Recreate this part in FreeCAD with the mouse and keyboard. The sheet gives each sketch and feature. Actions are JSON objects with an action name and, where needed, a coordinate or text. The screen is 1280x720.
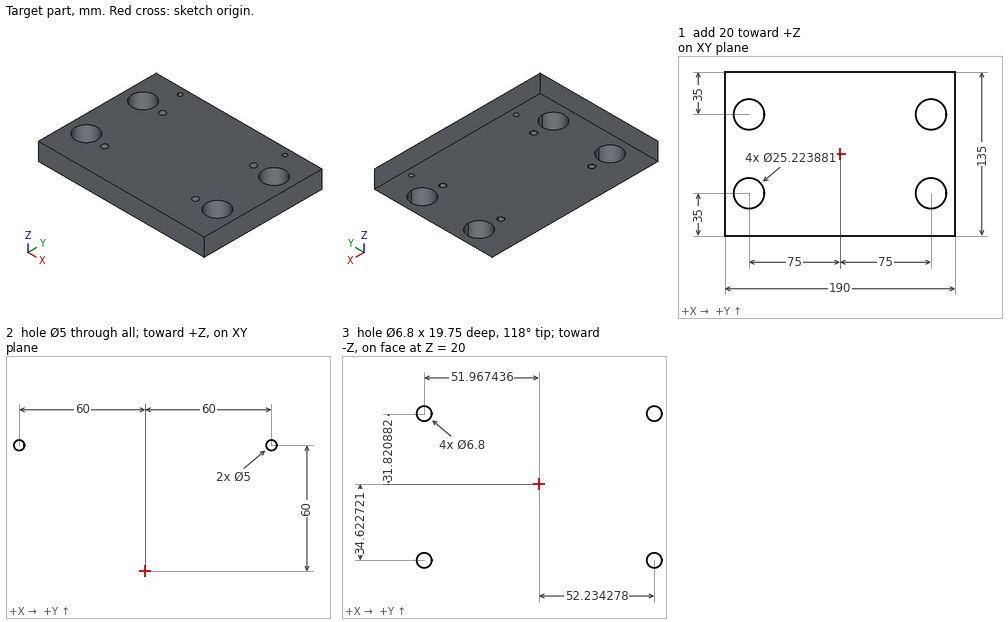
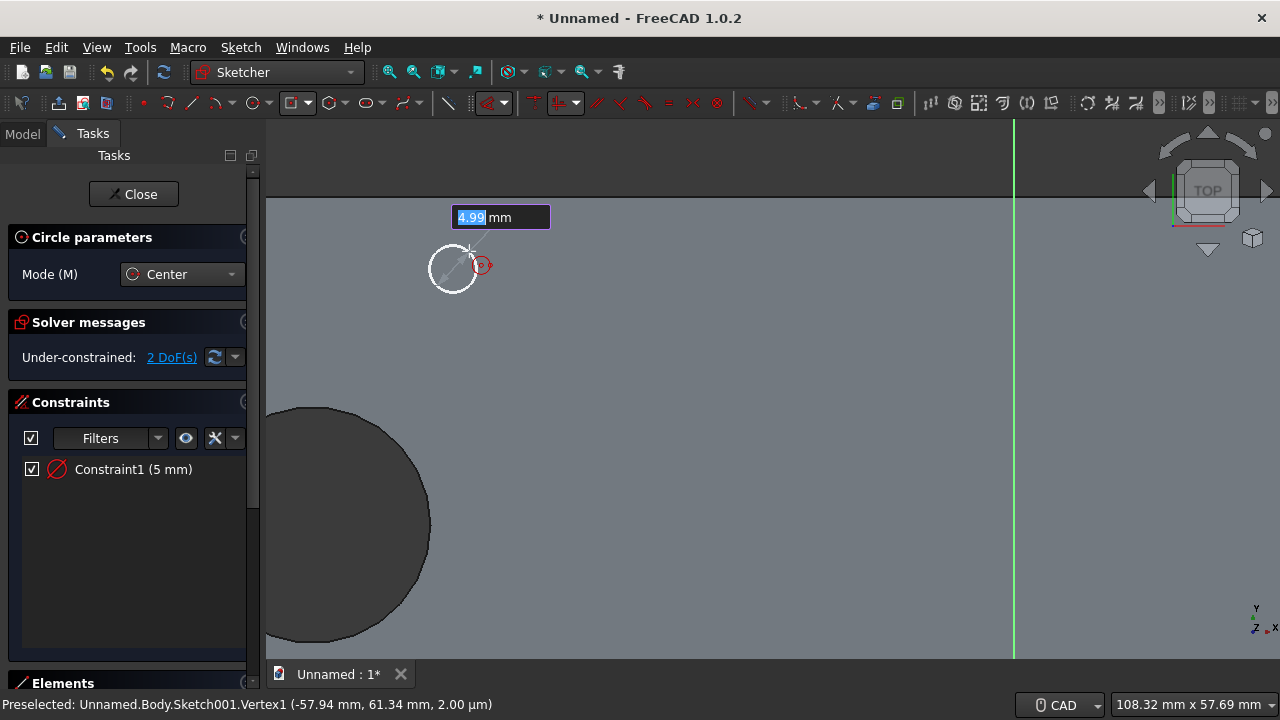
{"action": "type", "text": "5"}
{"action": "key", "text": "Return"}
{"action": "key", "text": "Escape"}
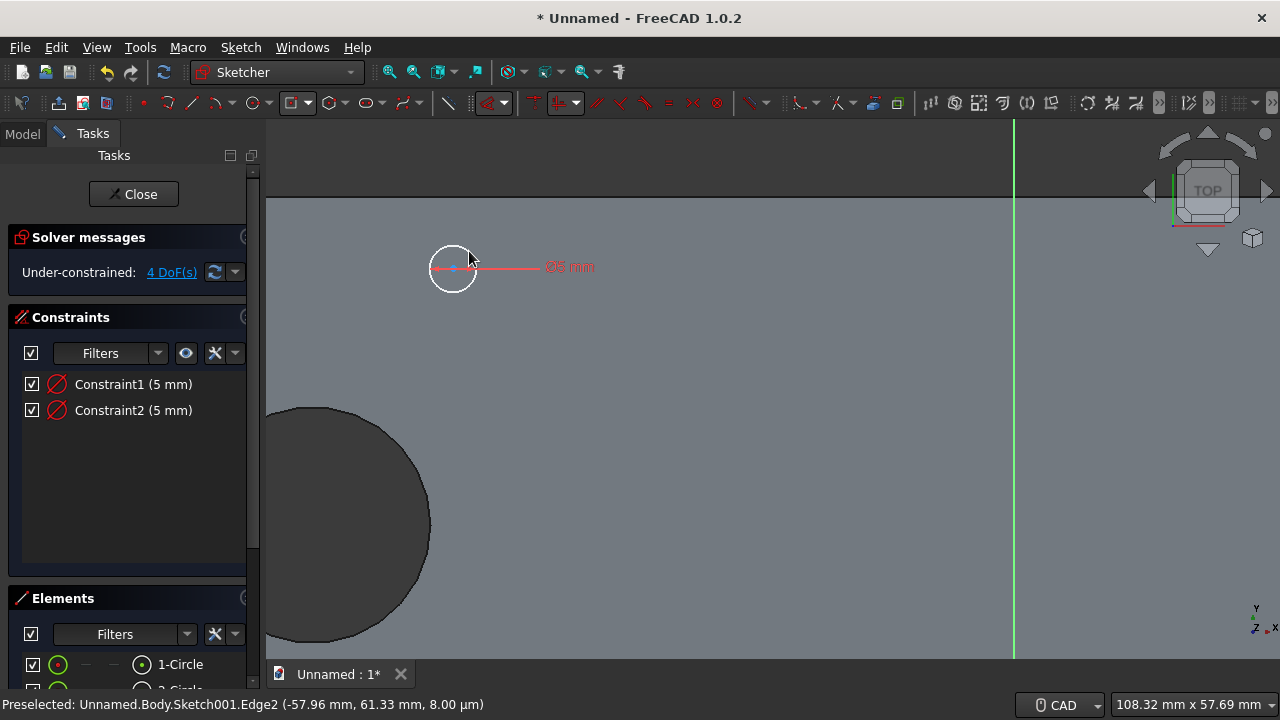
{"action": "scroll", "coordinate": [452, 268], "scroll_direction": "down", "scroll_amount": 4}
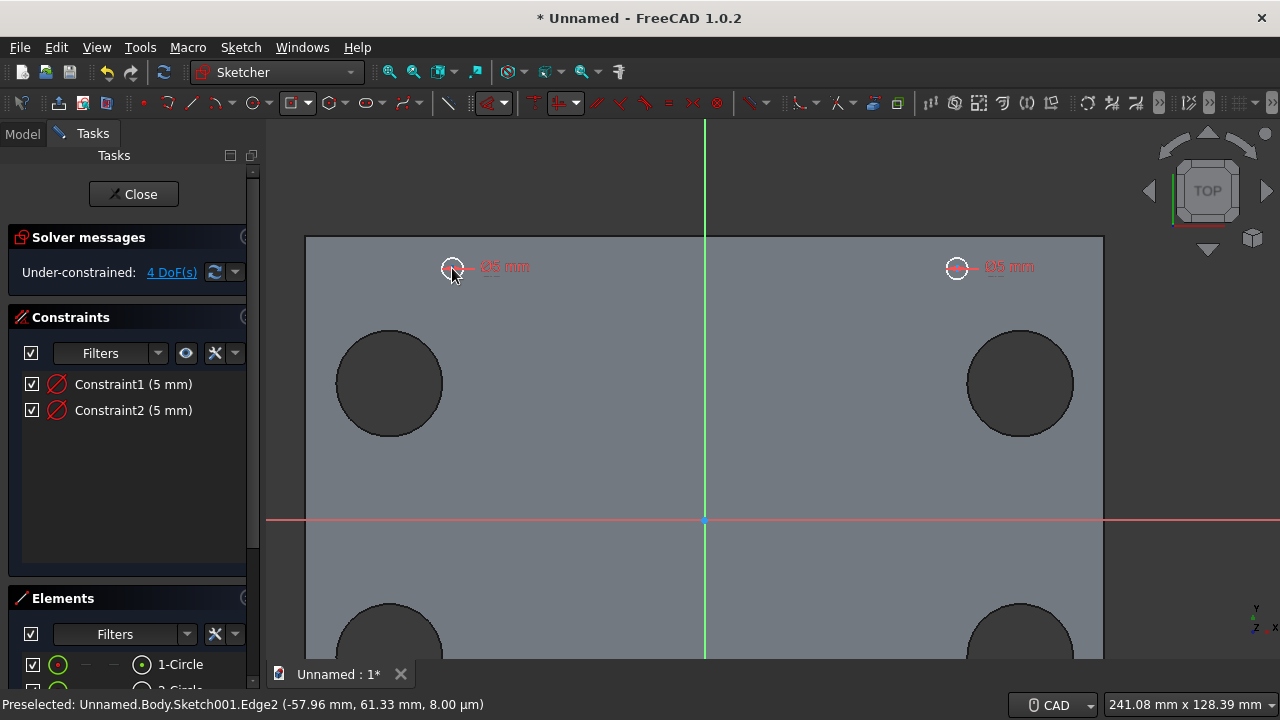
{"action": "left_click", "coordinate": [957, 269]}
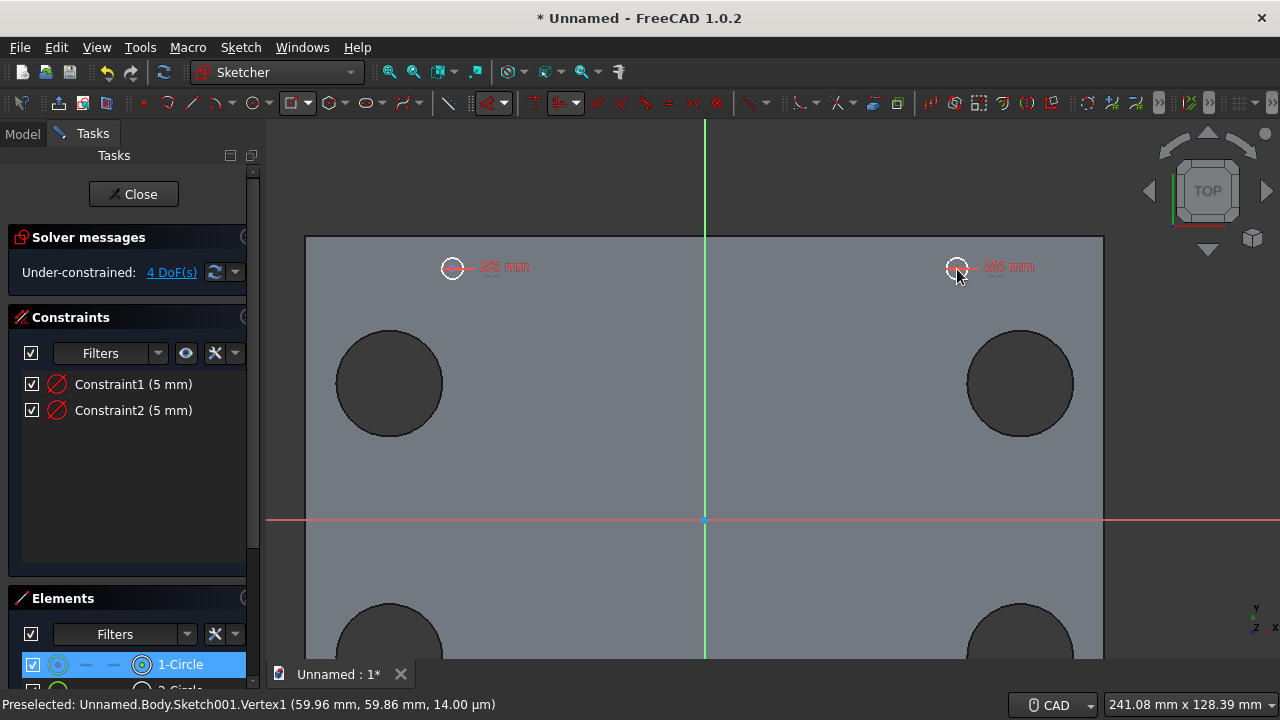
{"action": "left_click", "coordinate": [453, 269]}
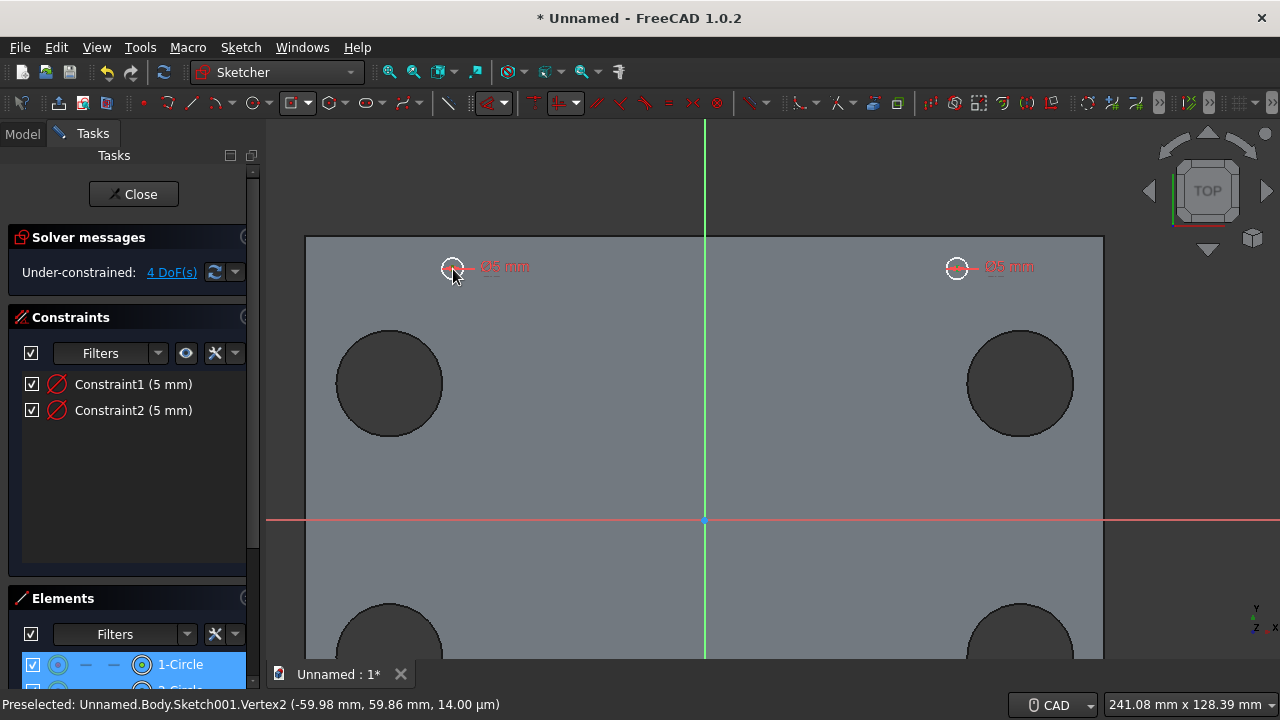
{"action": "key", "text": "h"}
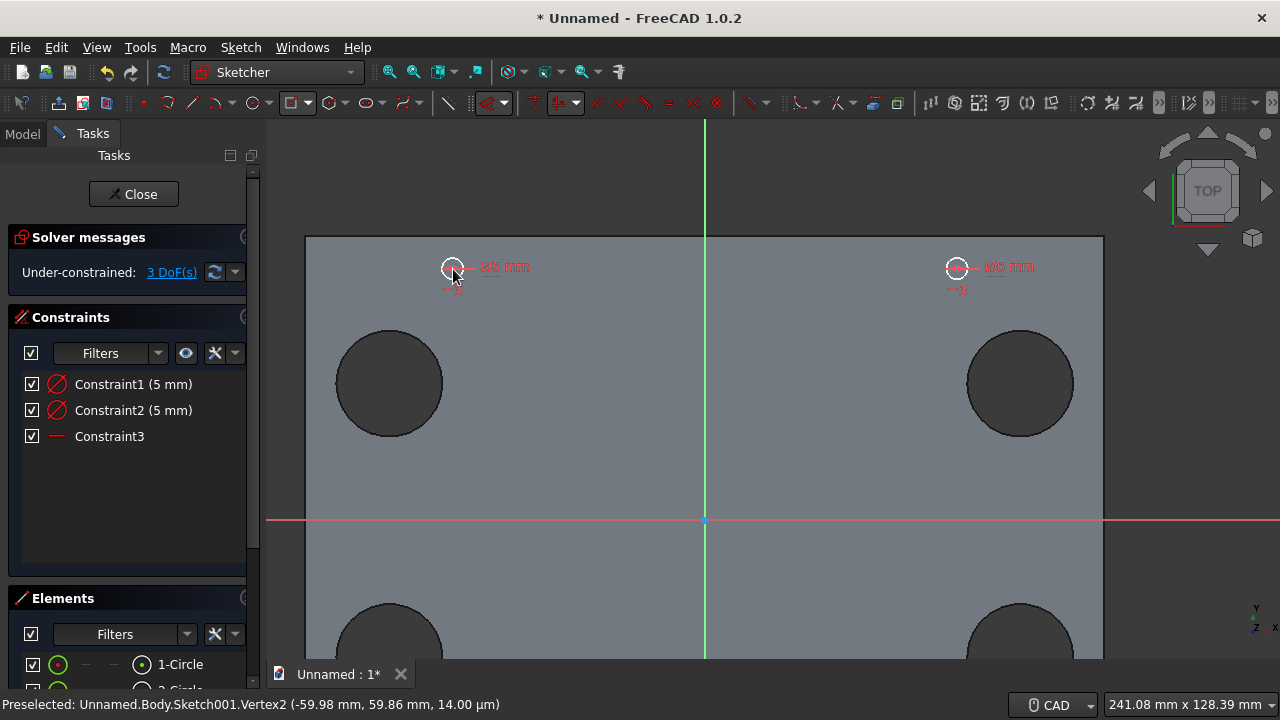
{"action": "left_click", "coordinate": [957, 269]}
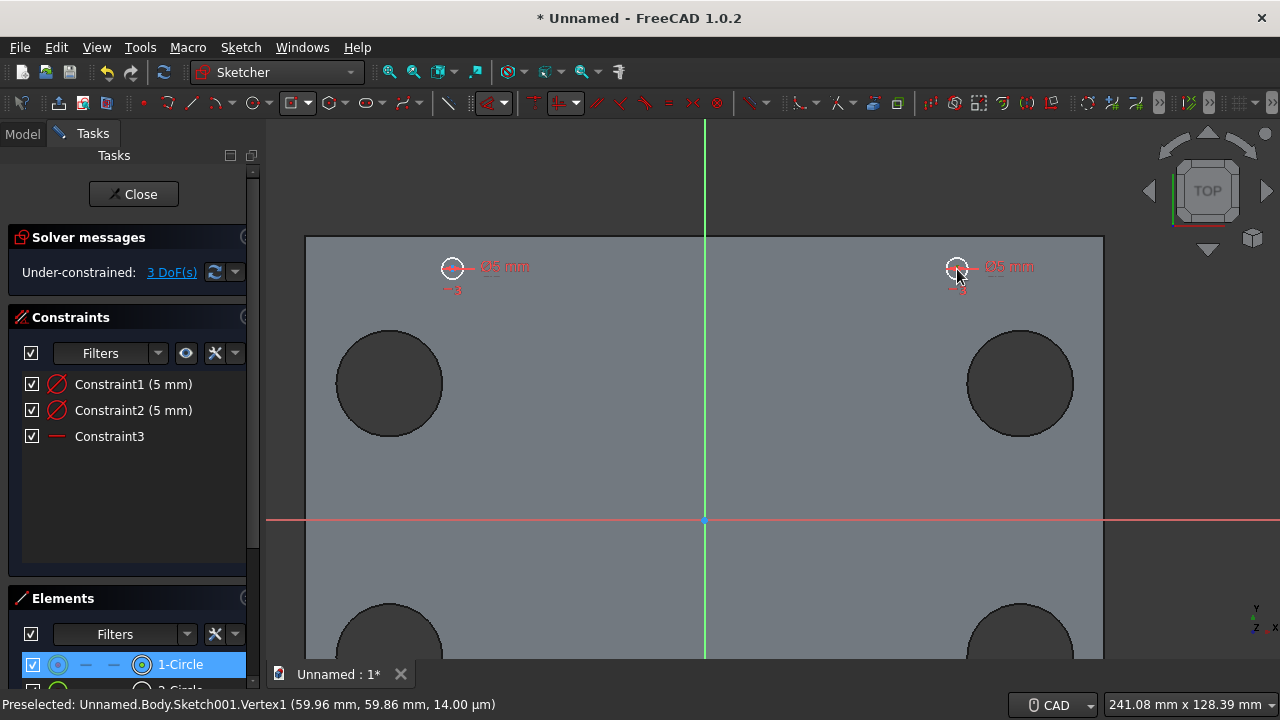
{"action": "key", "text": "l"}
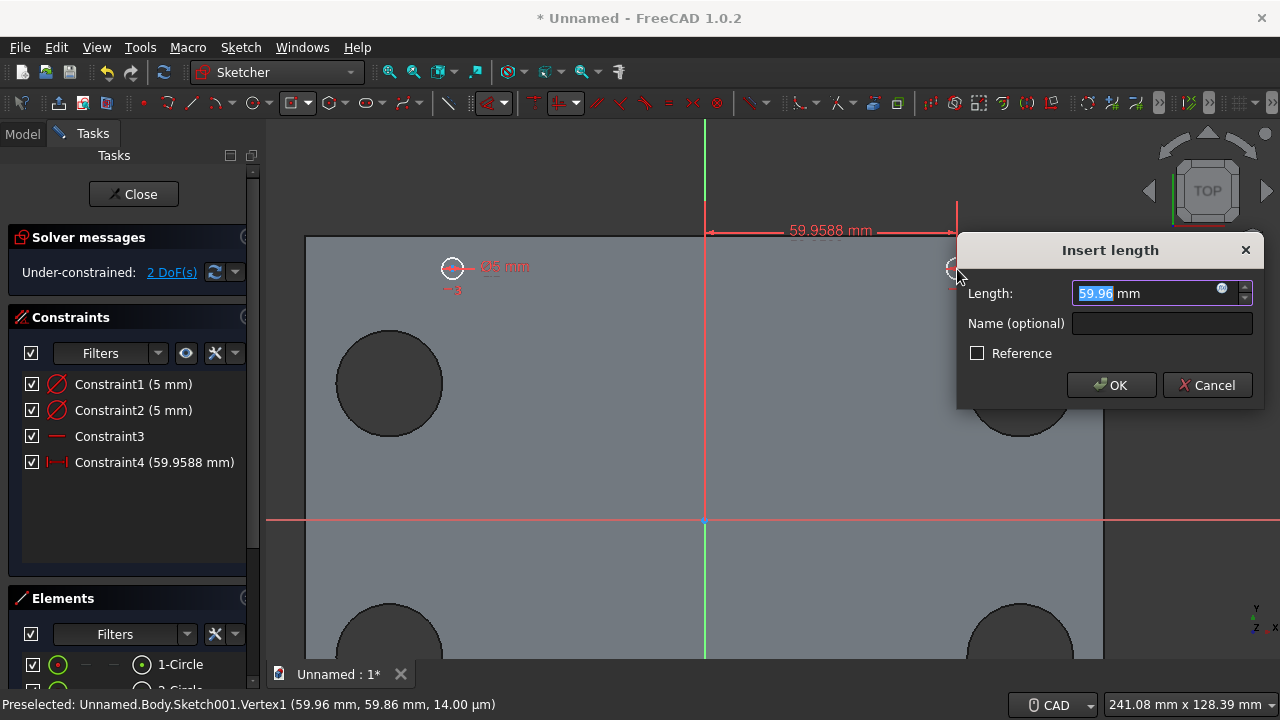
{"action": "type", "text": "60"}
{"action": "key", "text": "Return"}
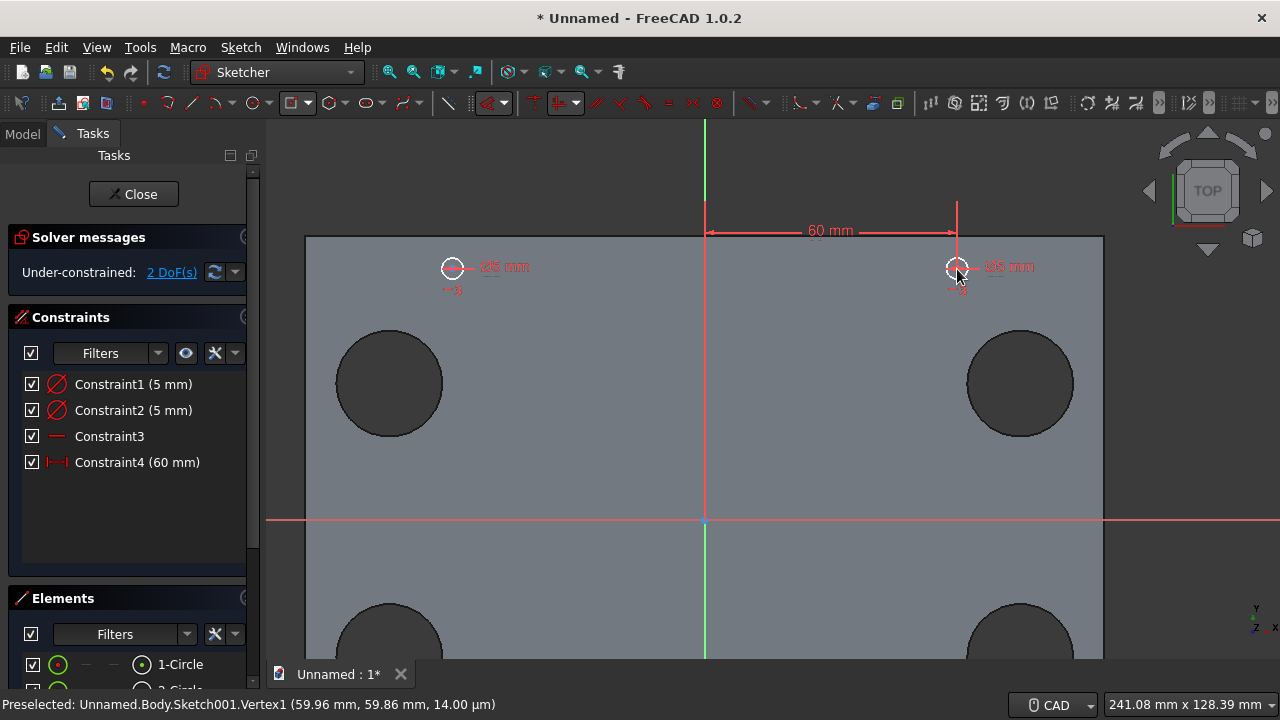
{"action": "left_click", "coordinate": [957, 269]}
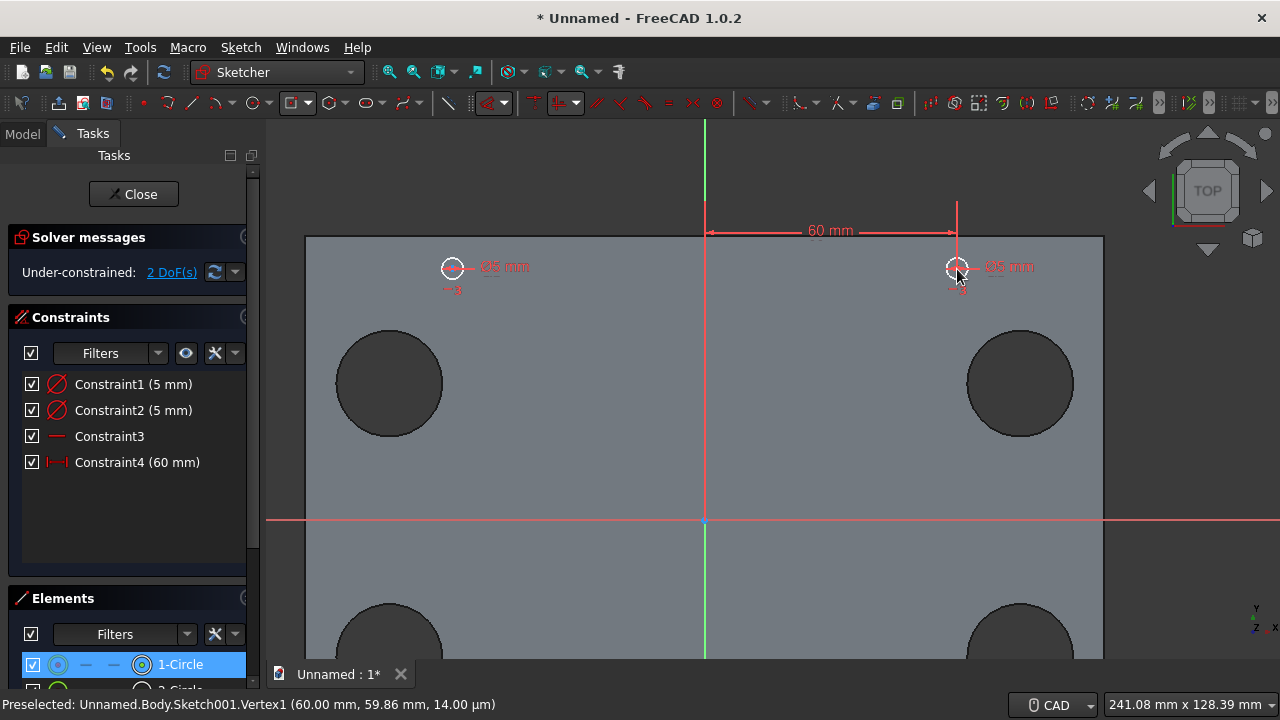
{"action": "left_click", "coordinate": [506, 104]}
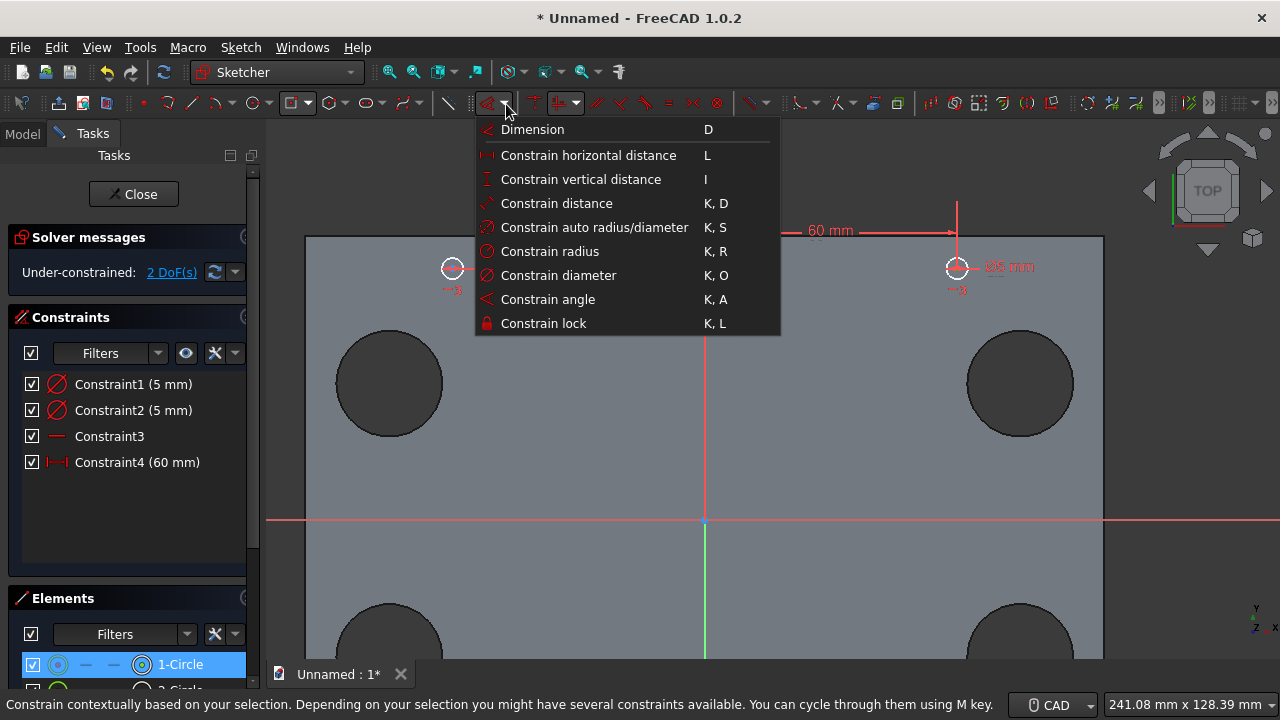
{"action": "left_click", "coordinate": [628, 179]}